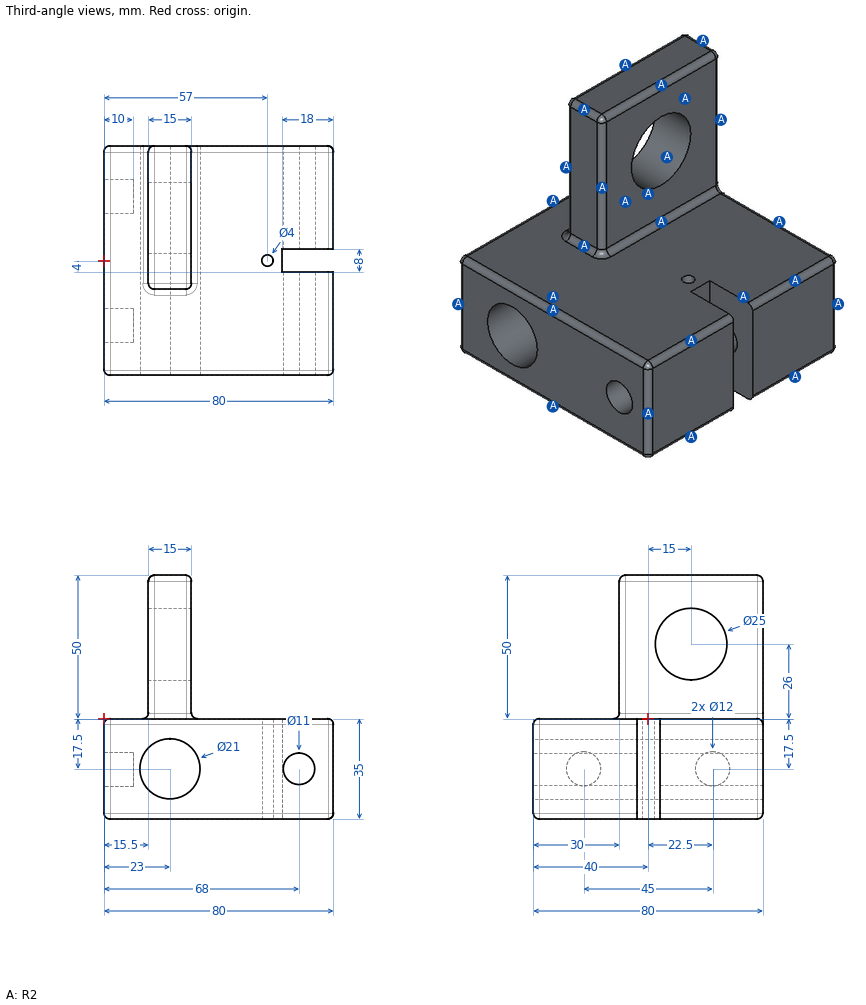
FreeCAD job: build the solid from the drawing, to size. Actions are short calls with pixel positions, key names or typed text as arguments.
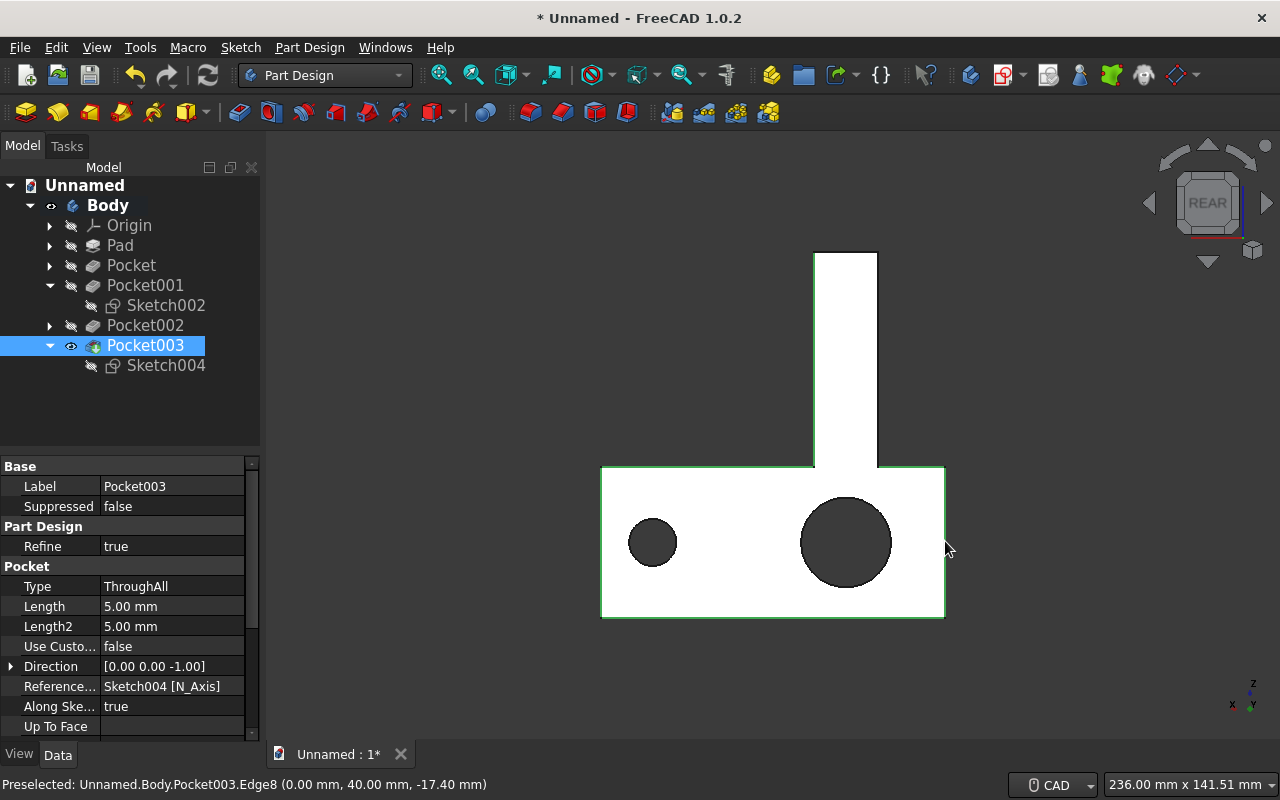
click(878, 359, ctrl)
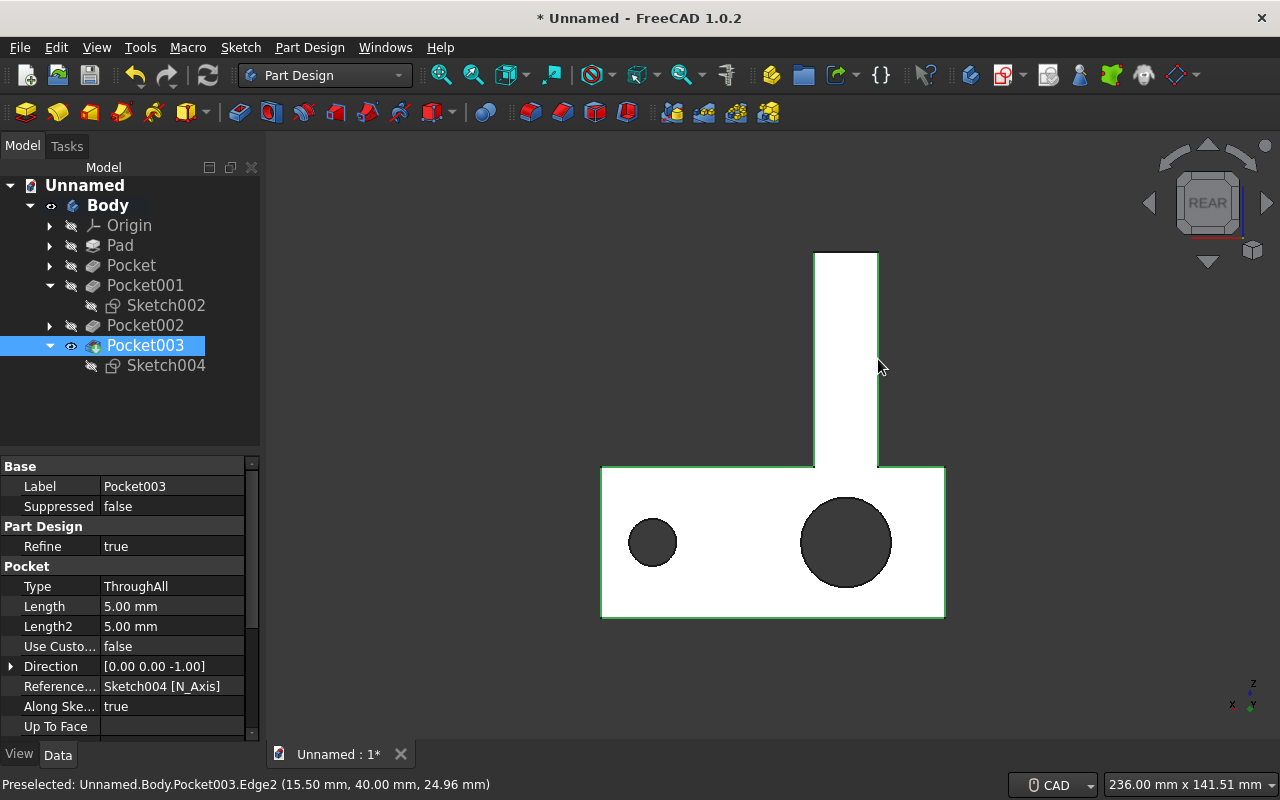
key(6)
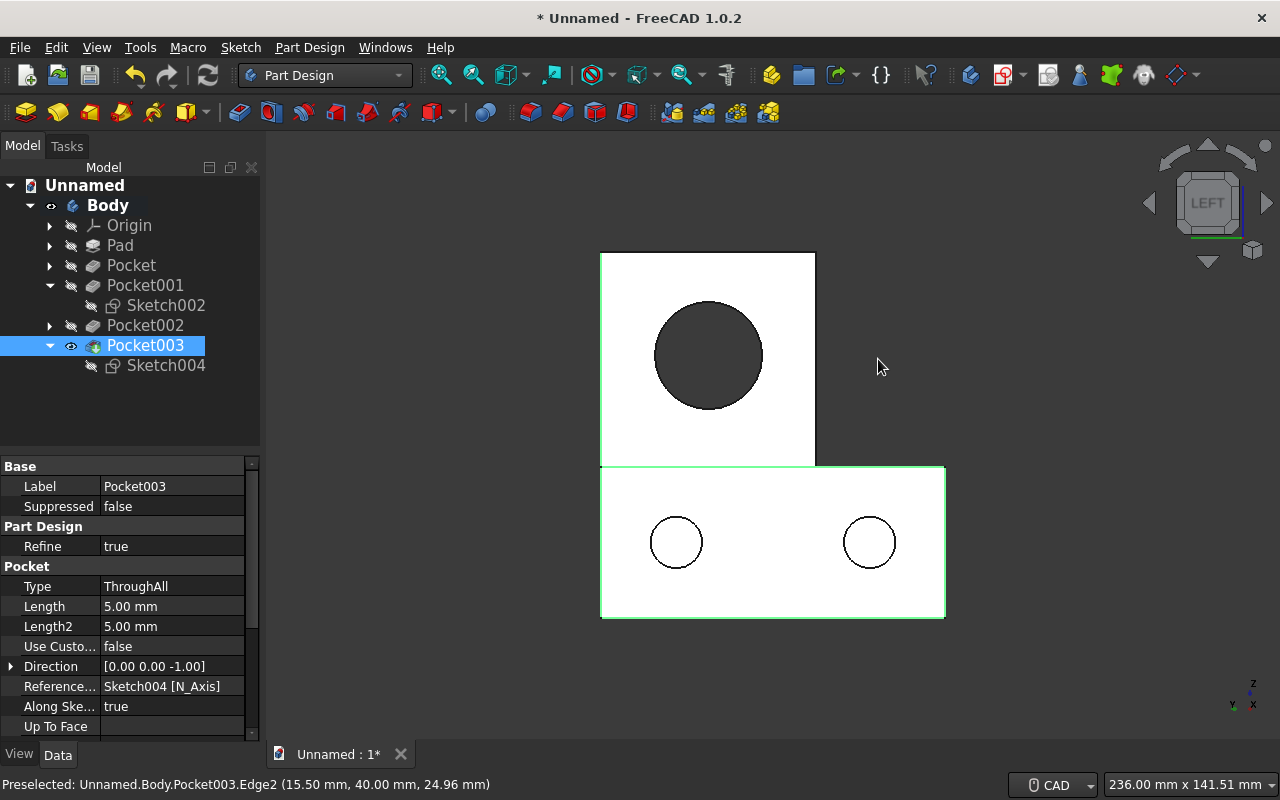
key(v)
key(3)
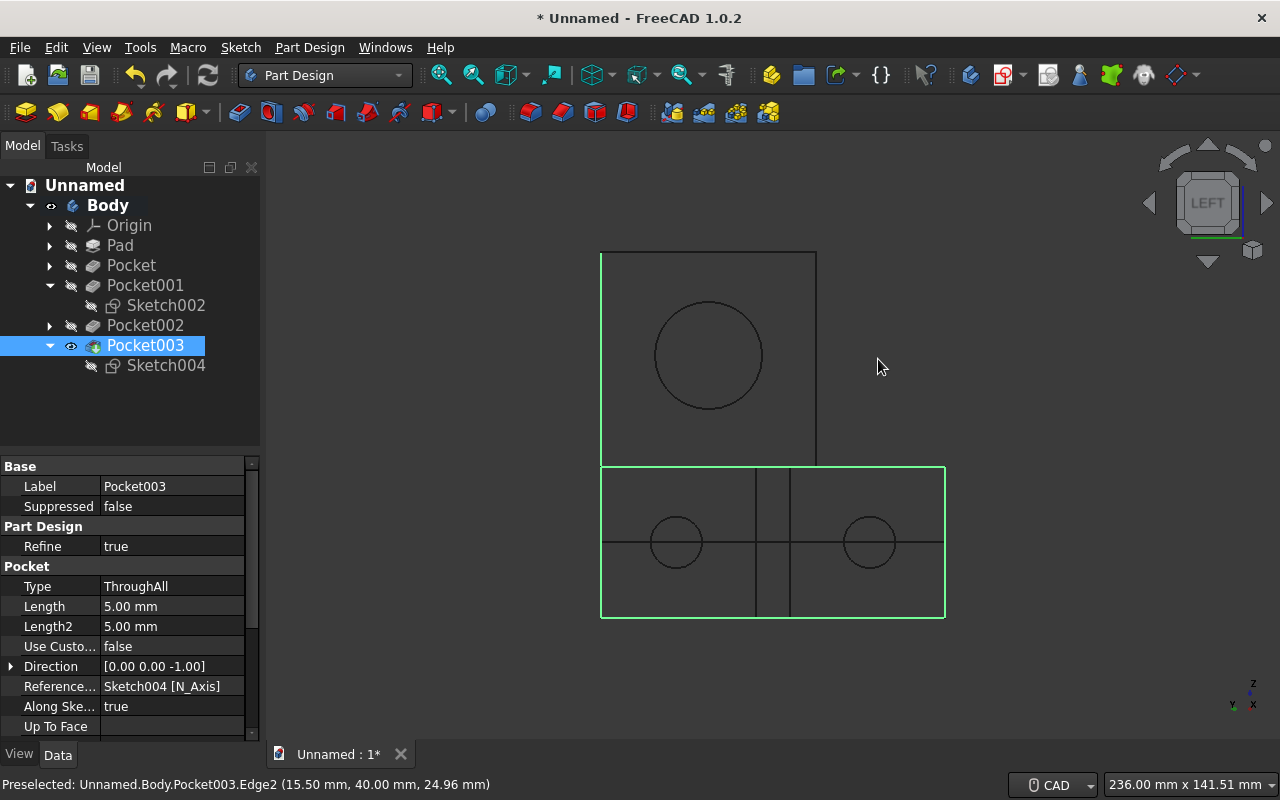
key(0)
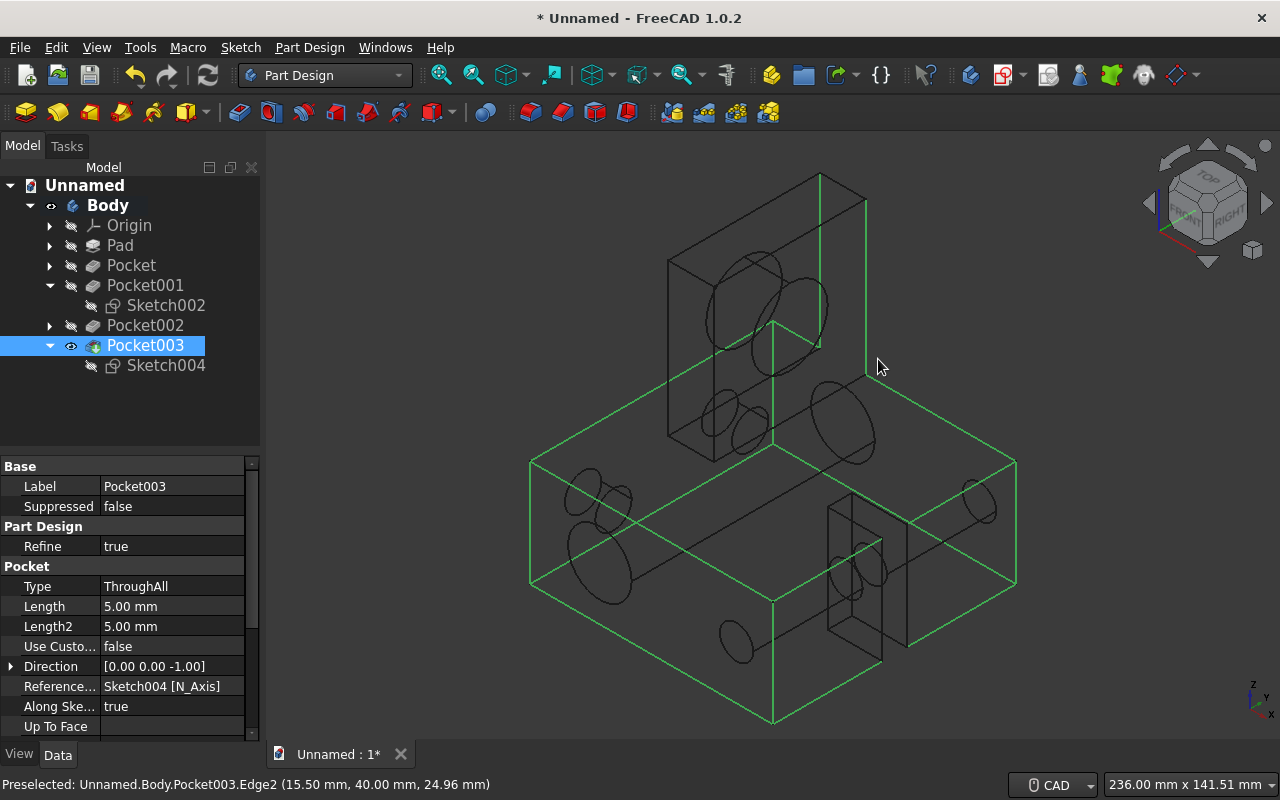
click(744, 391, ctrl)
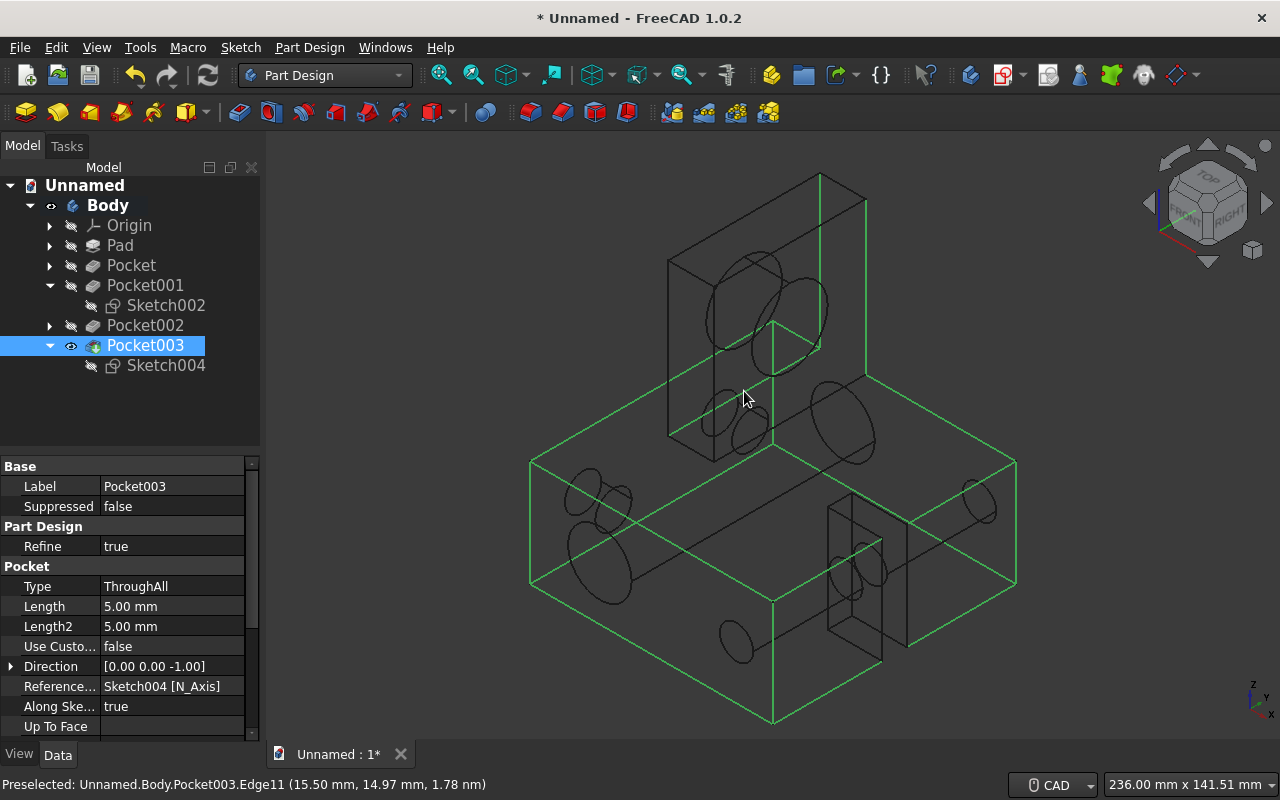
click(790, 417, ctrl)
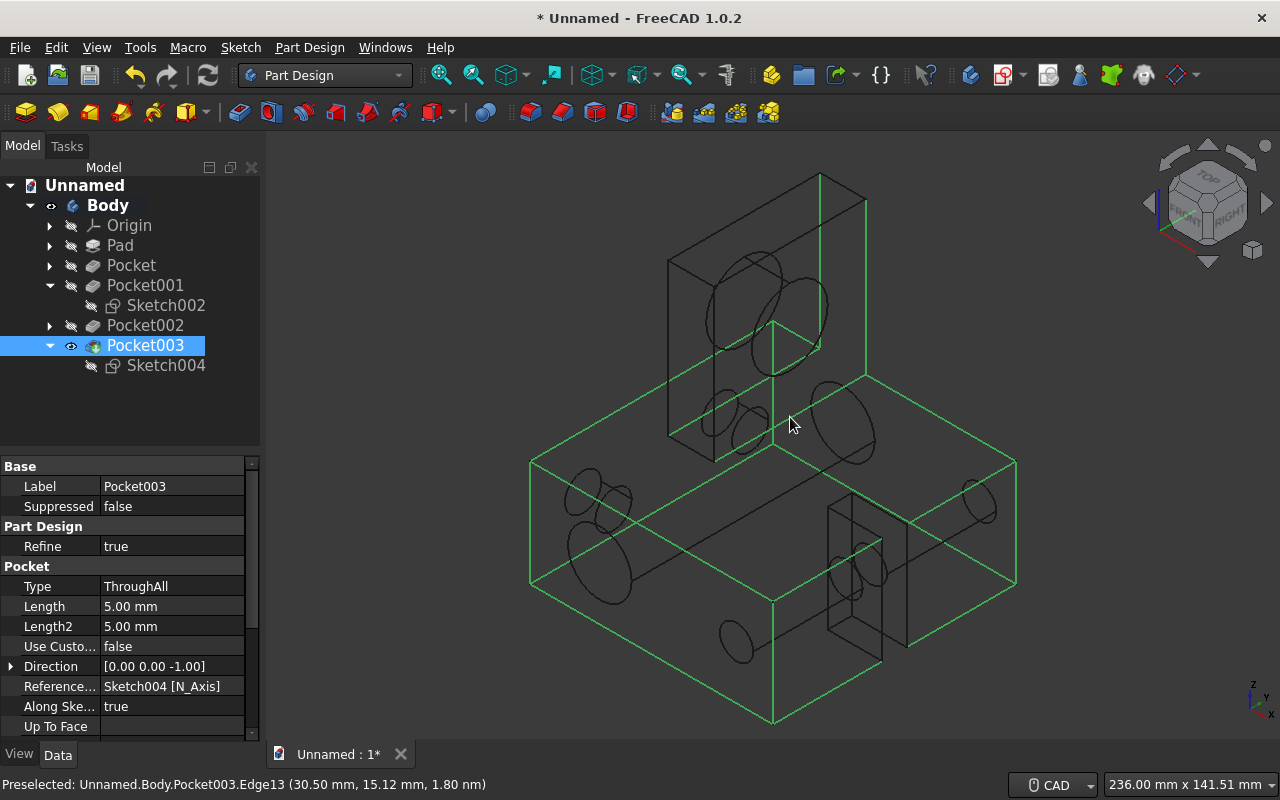
key(v)
key(1)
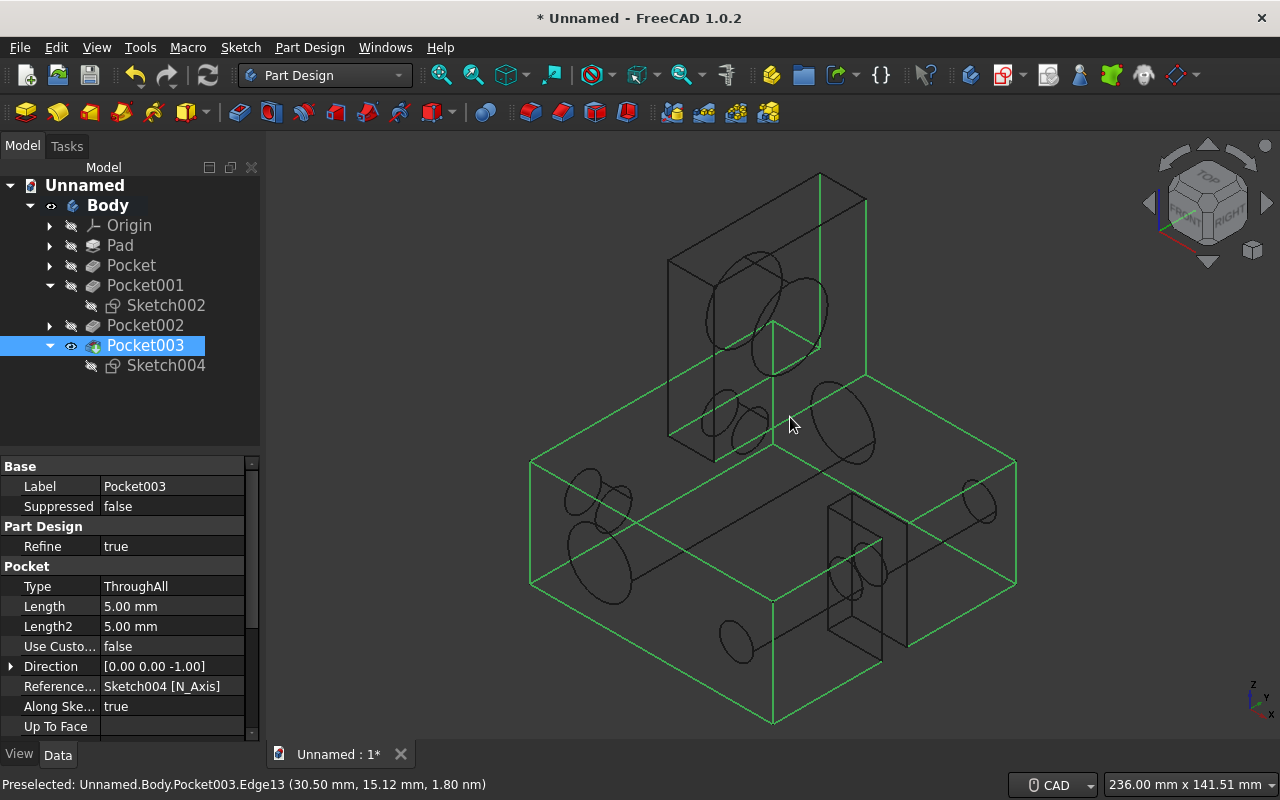
click(532, 112)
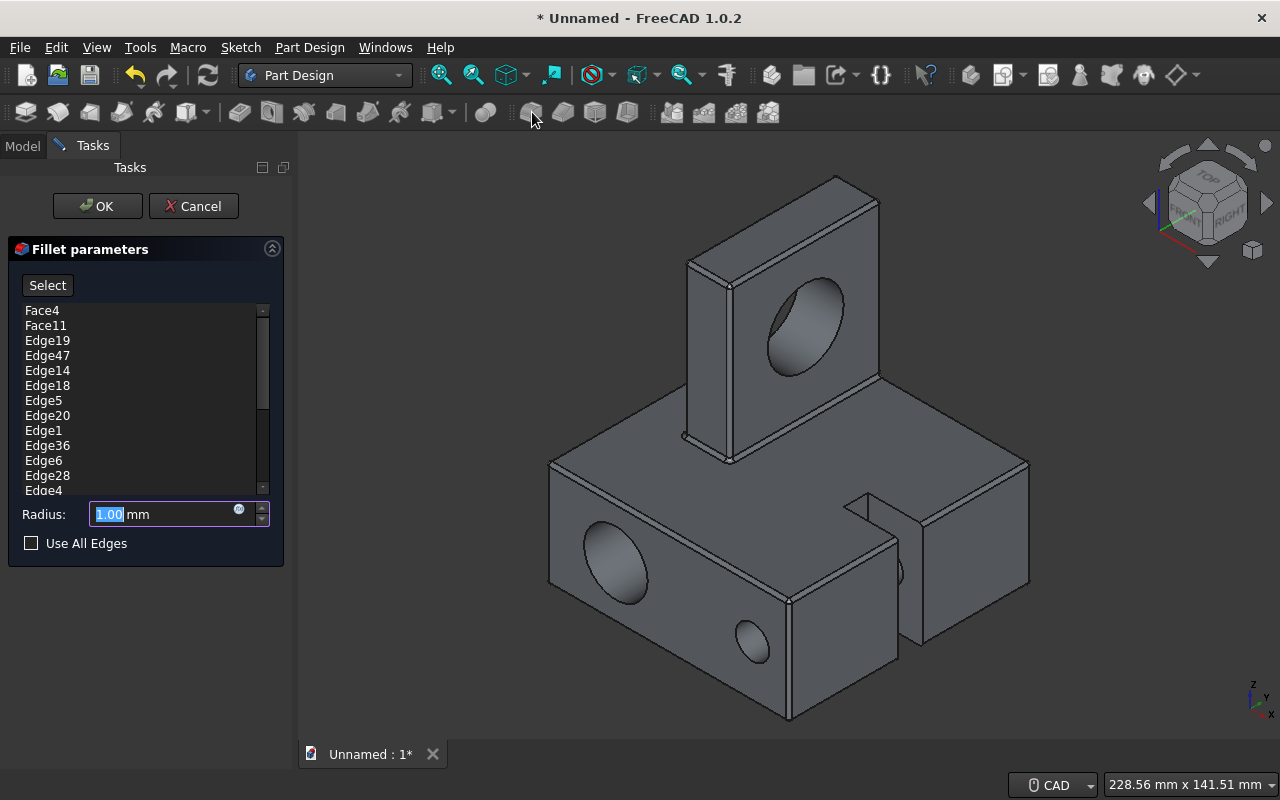
text(2)
key(Tab)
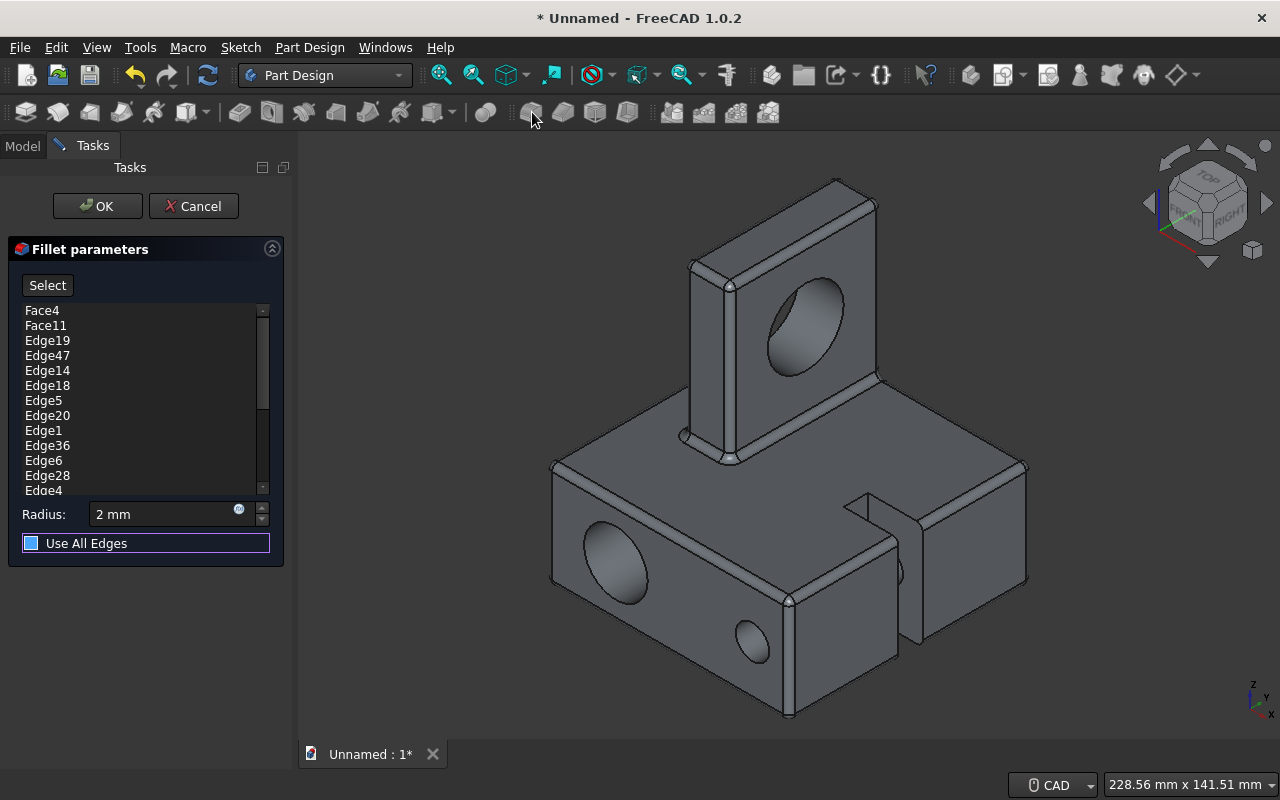
click(98, 206)